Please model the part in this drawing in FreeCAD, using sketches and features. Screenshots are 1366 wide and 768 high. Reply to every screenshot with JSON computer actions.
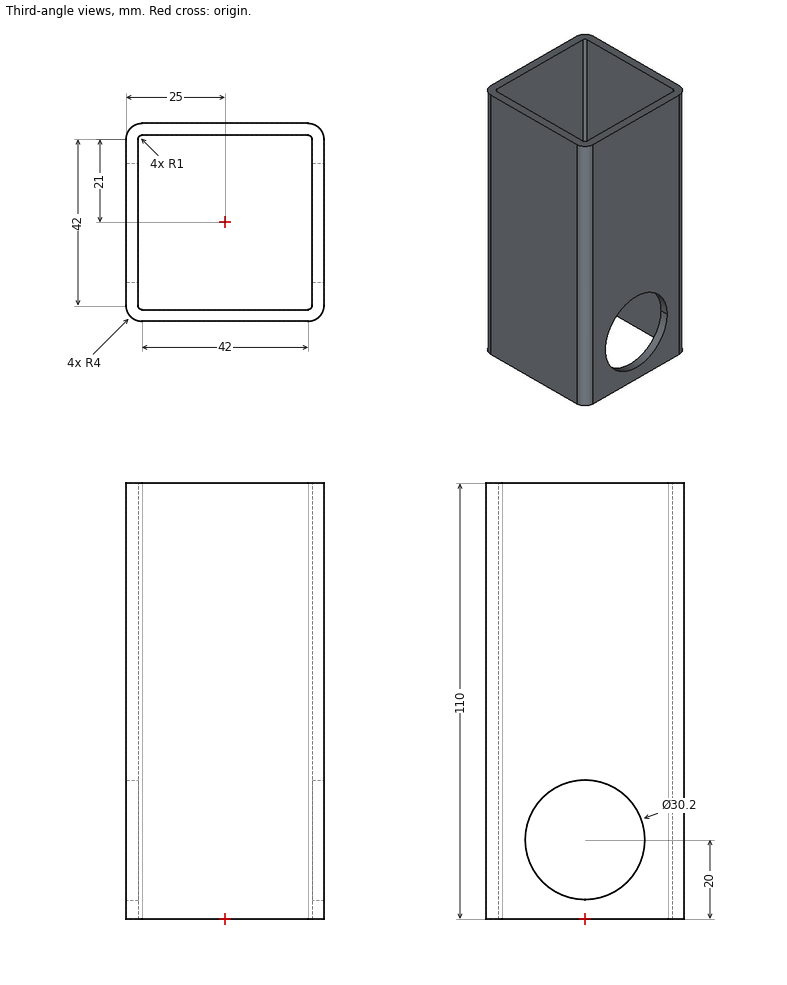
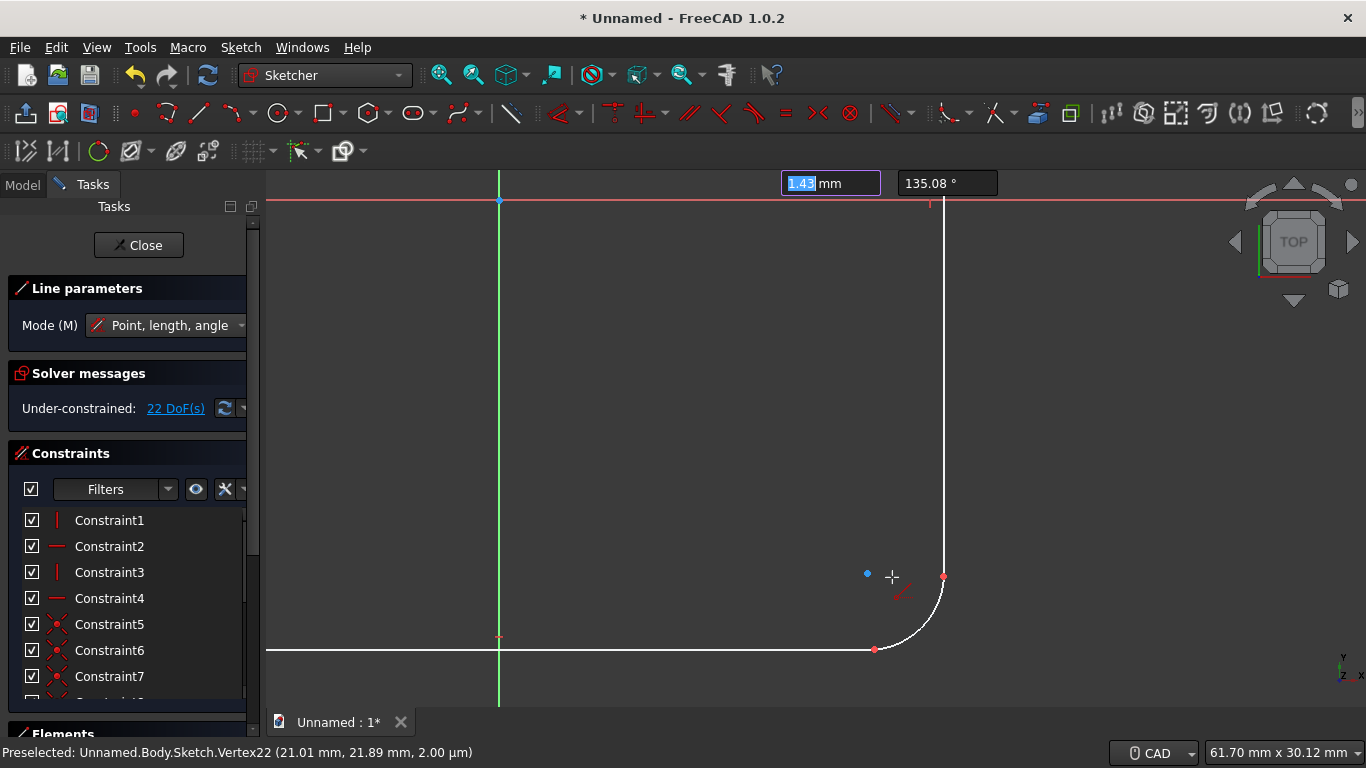
{"action": "left_click", "coordinate": [892, 574]}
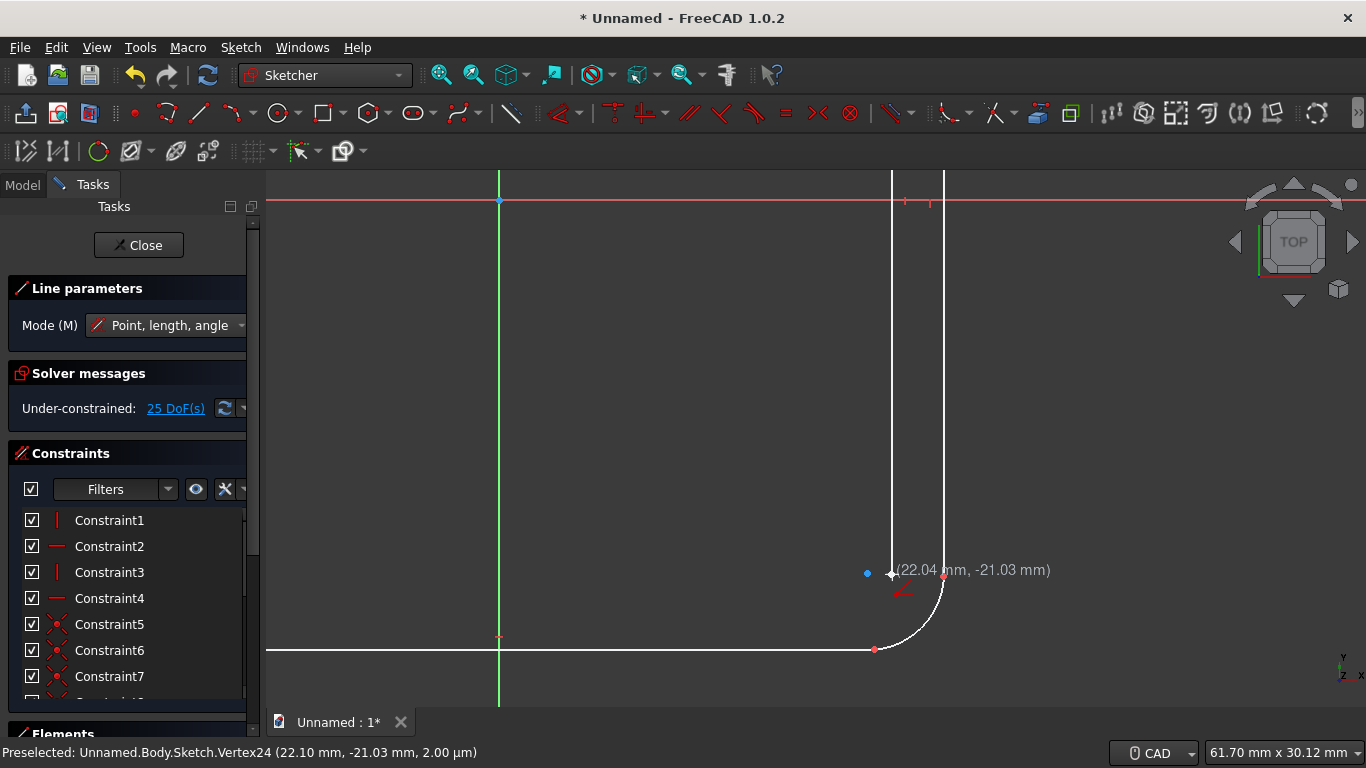
{"action": "left_click", "coordinate": [873, 592]}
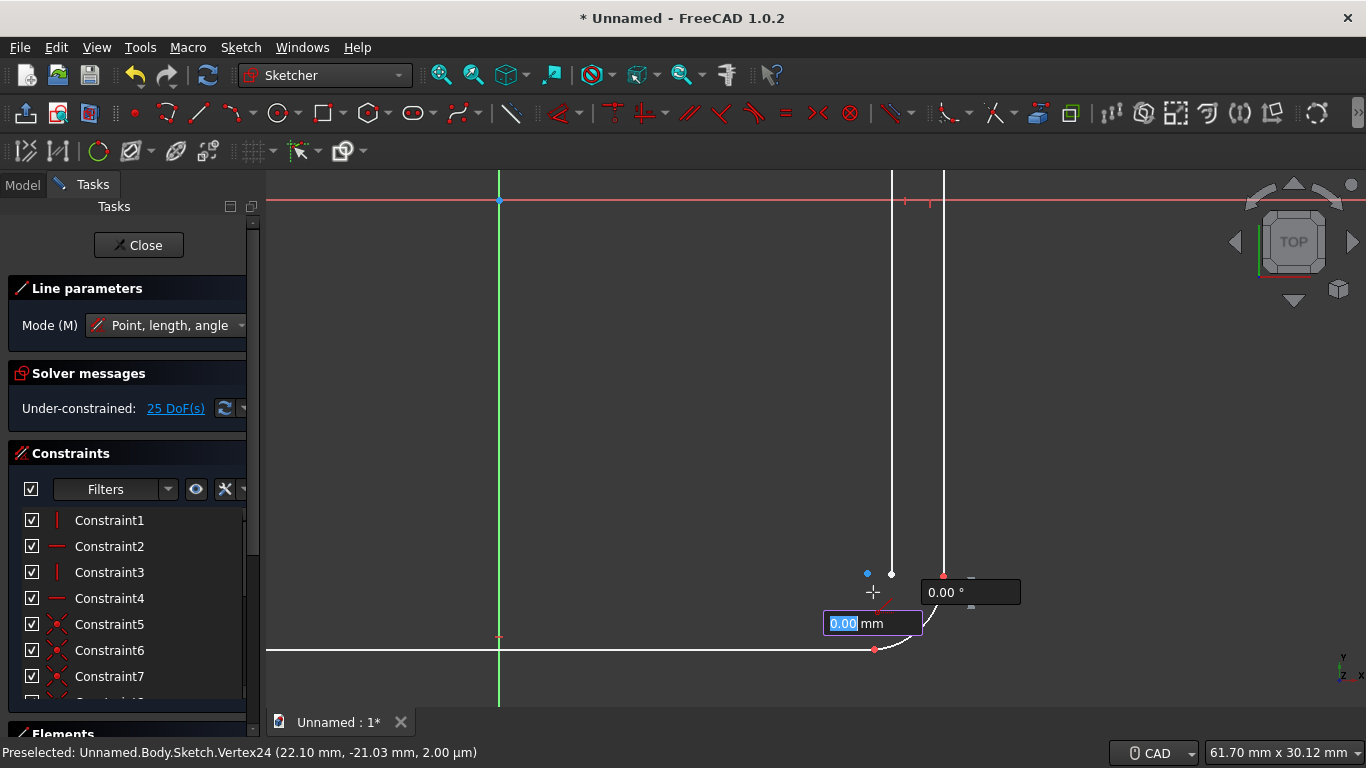
{"action": "scroll", "coordinate": [892, 577], "scroll_direction": "down", "scroll_amount": 5}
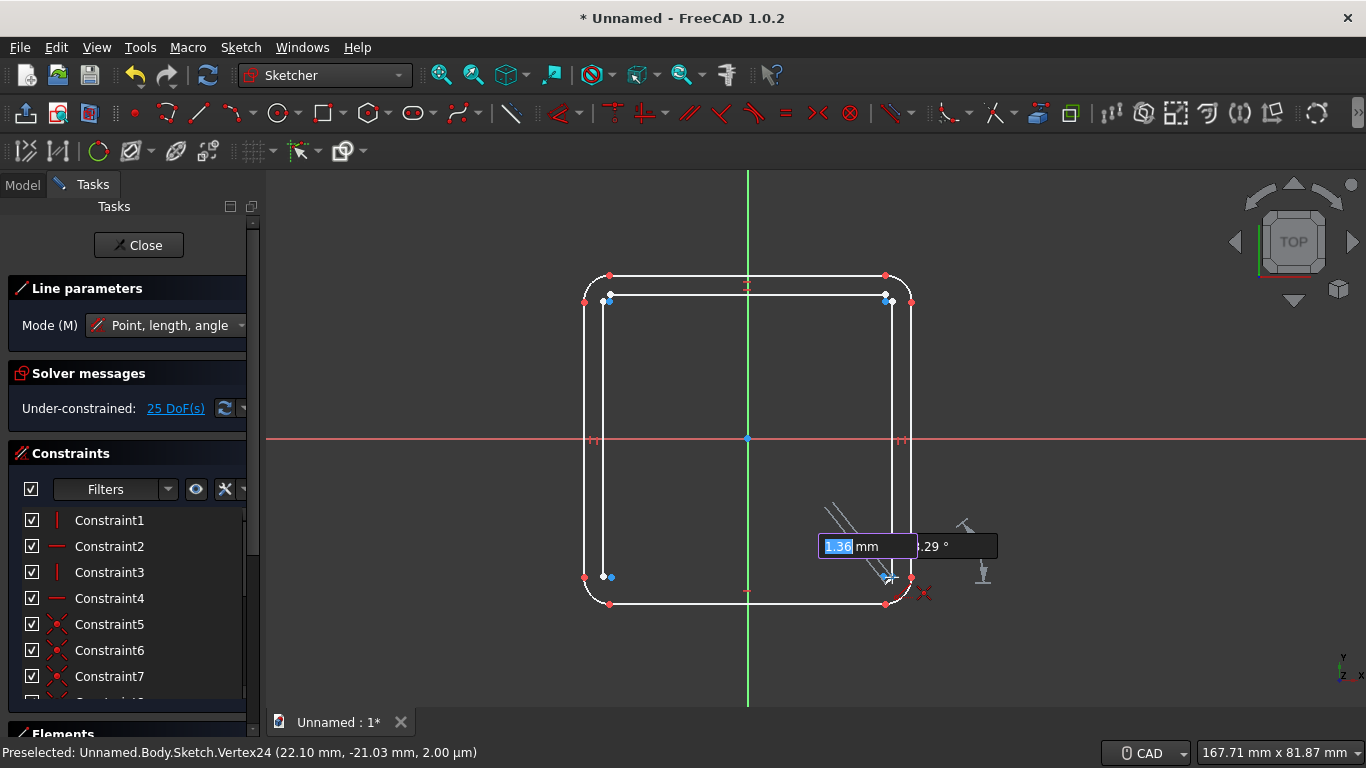
{"action": "scroll", "coordinate": [610, 583], "scroll_direction": "up", "scroll_amount": 5}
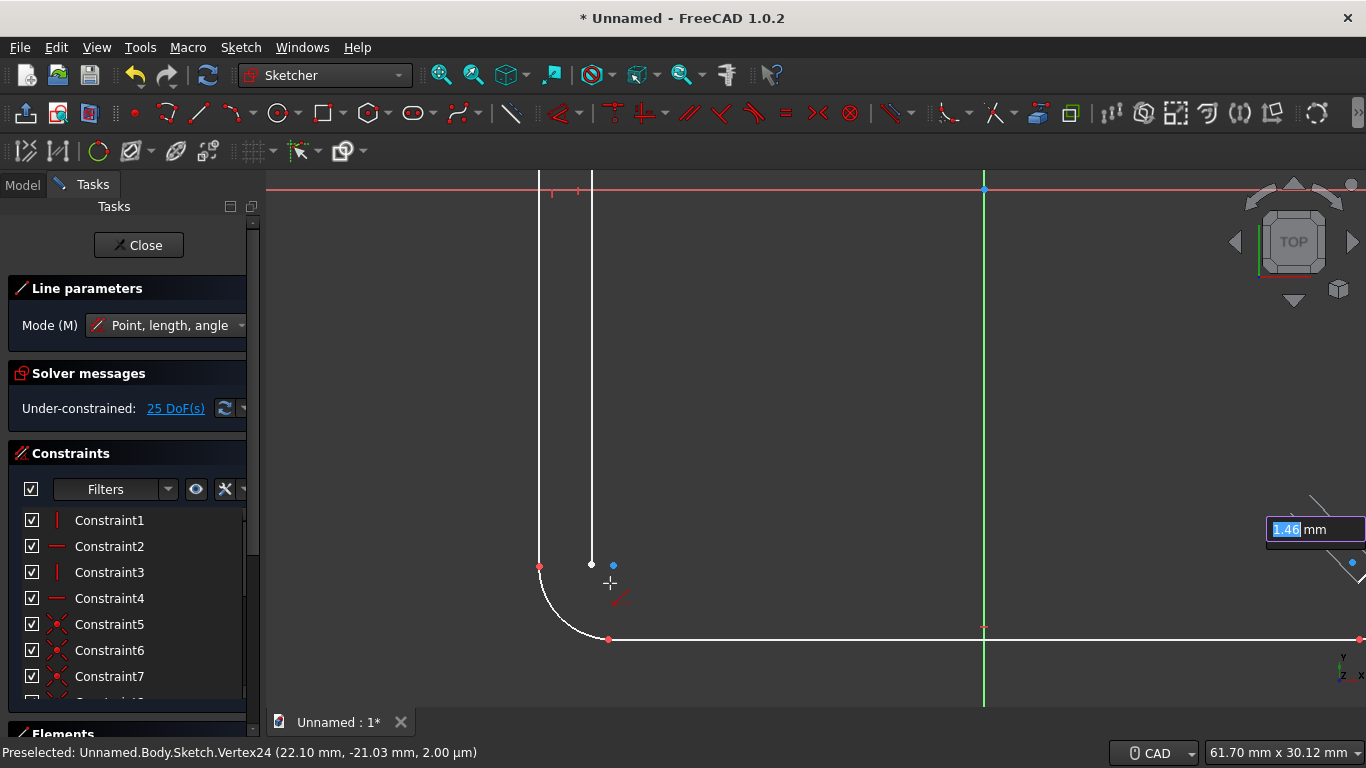
{"action": "left_click", "coordinate": [610, 582]}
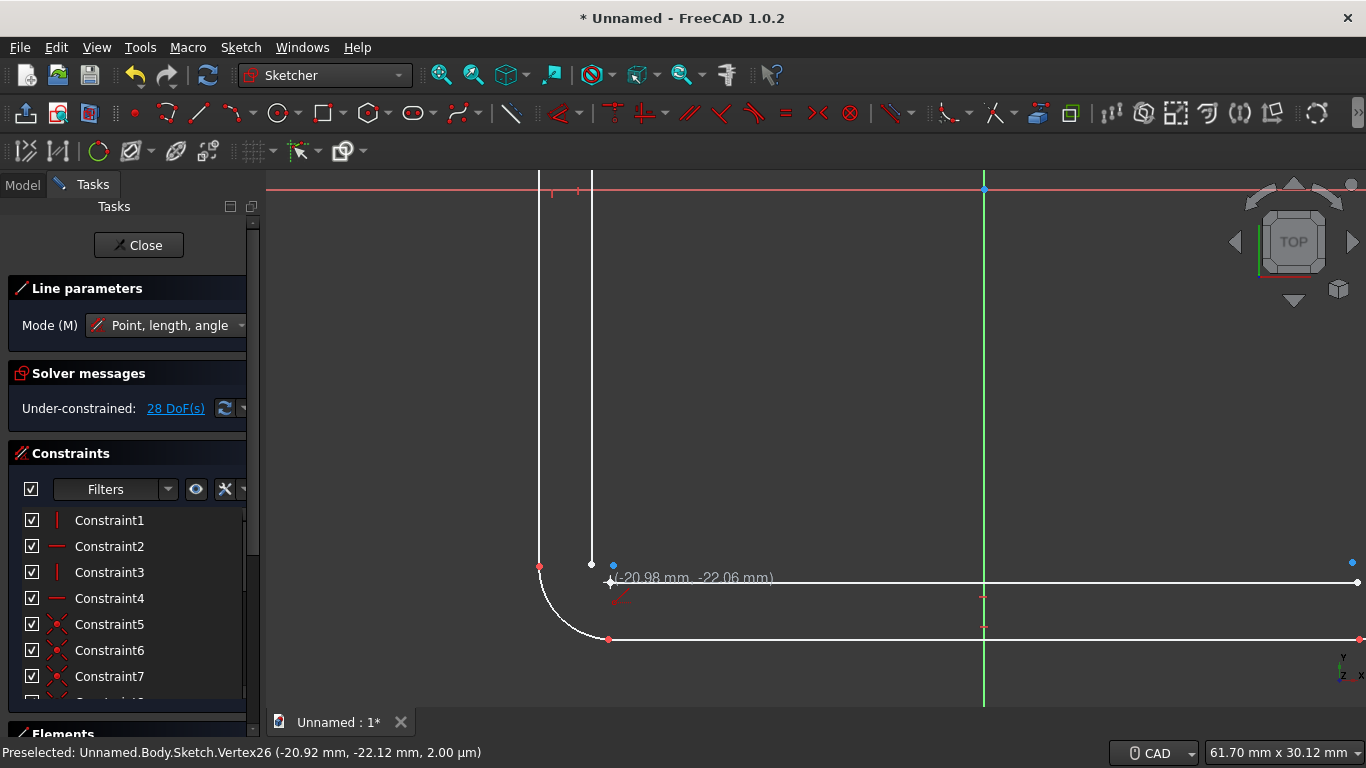
{"action": "left_click", "coordinate": [232, 114]}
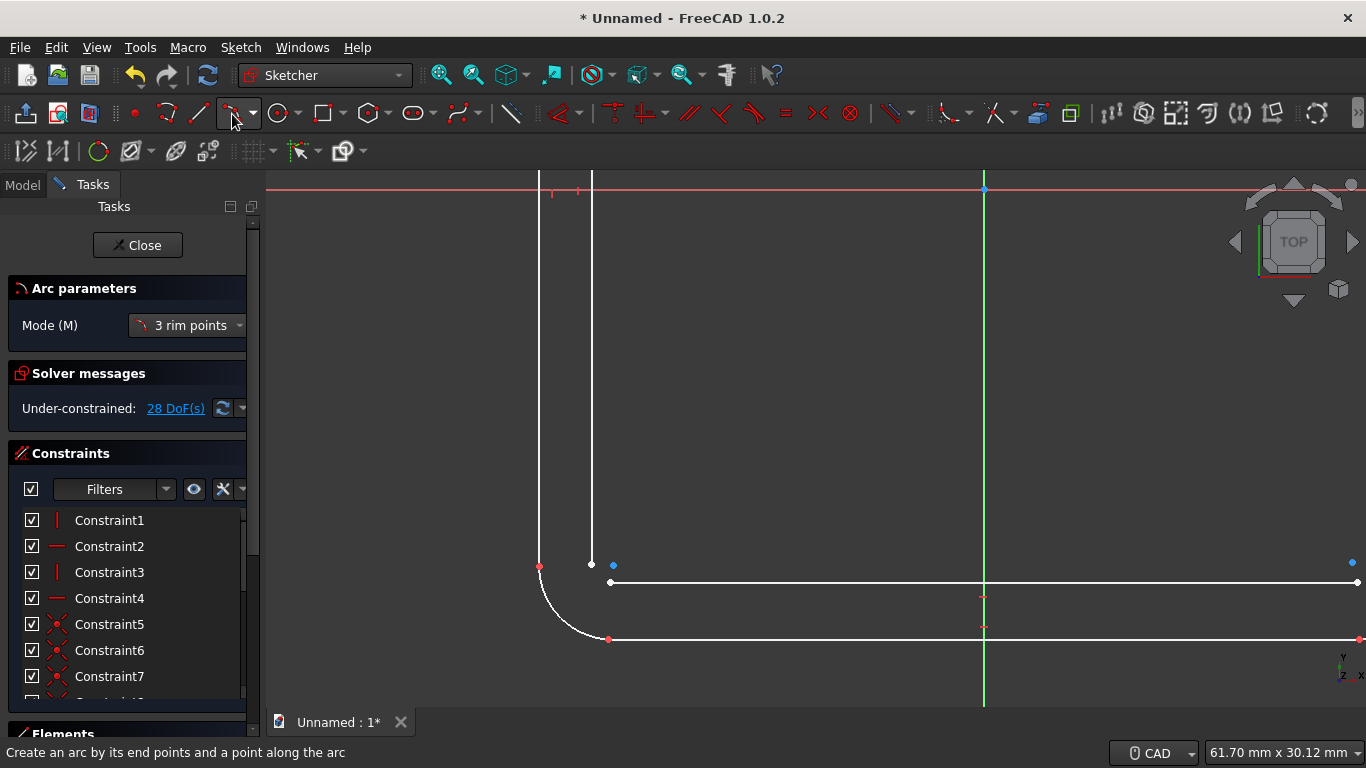
{"action": "scroll", "coordinate": [610, 583], "scroll_direction": "down", "scroll_amount": 5}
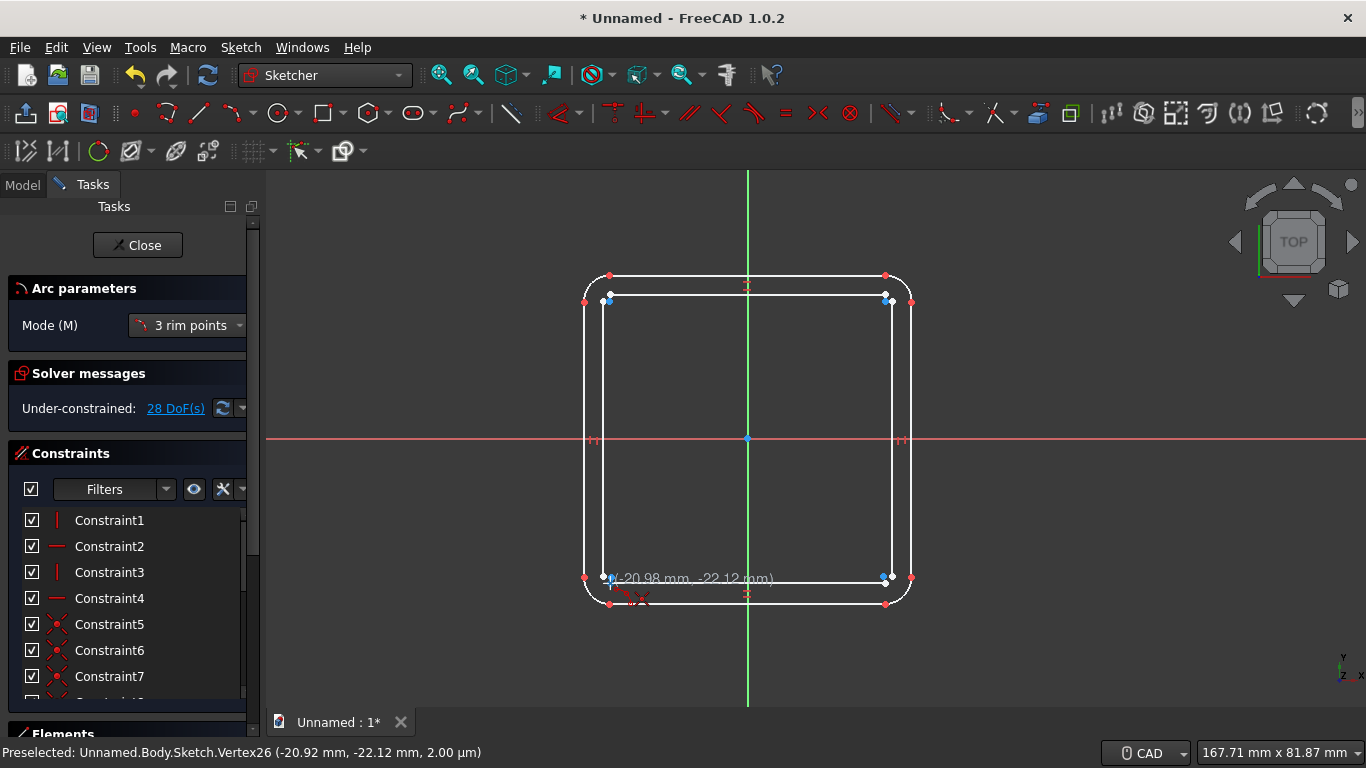
{"action": "scroll", "coordinate": [604, 301], "scroll_direction": "up", "scroll_amount": 5}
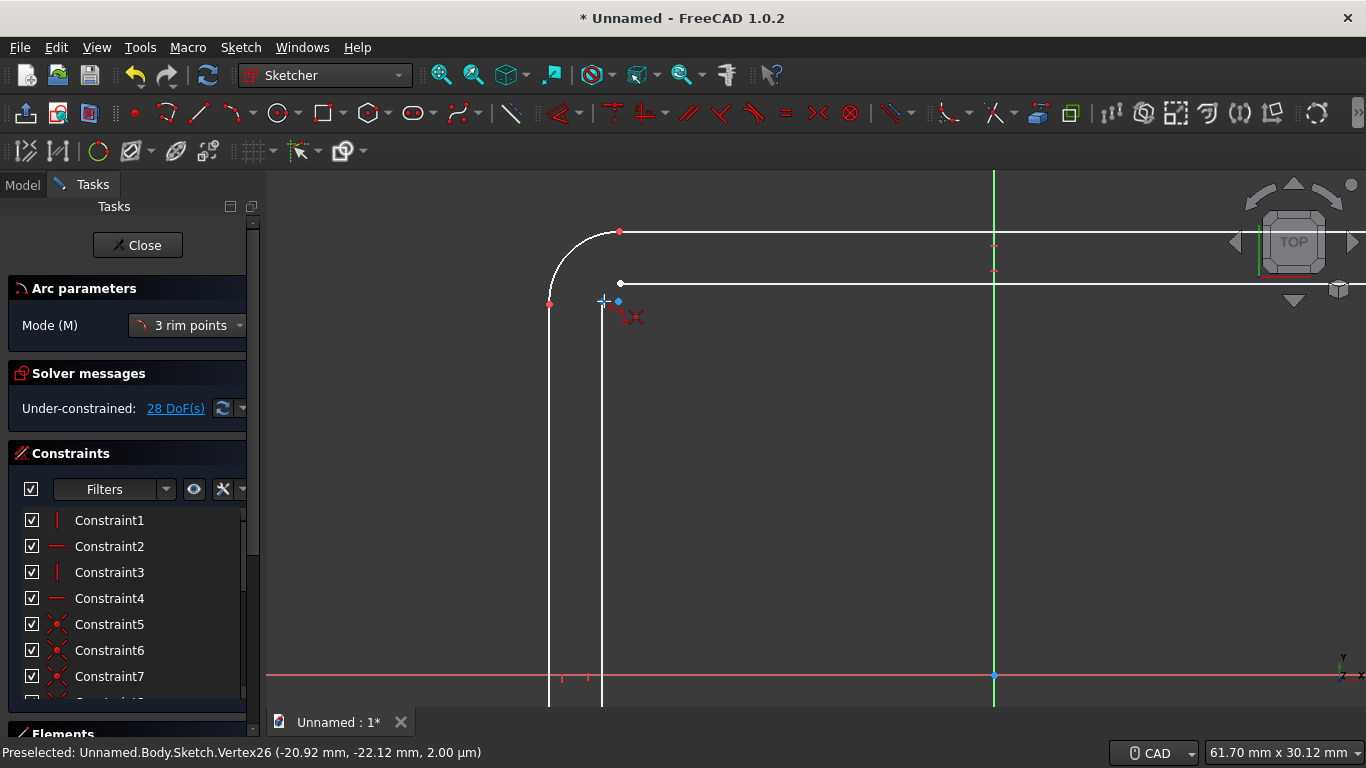
{"action": "left_click", "coordinate": [602, 302]}
{"action": "left_click", "coordinate": [620, 284]}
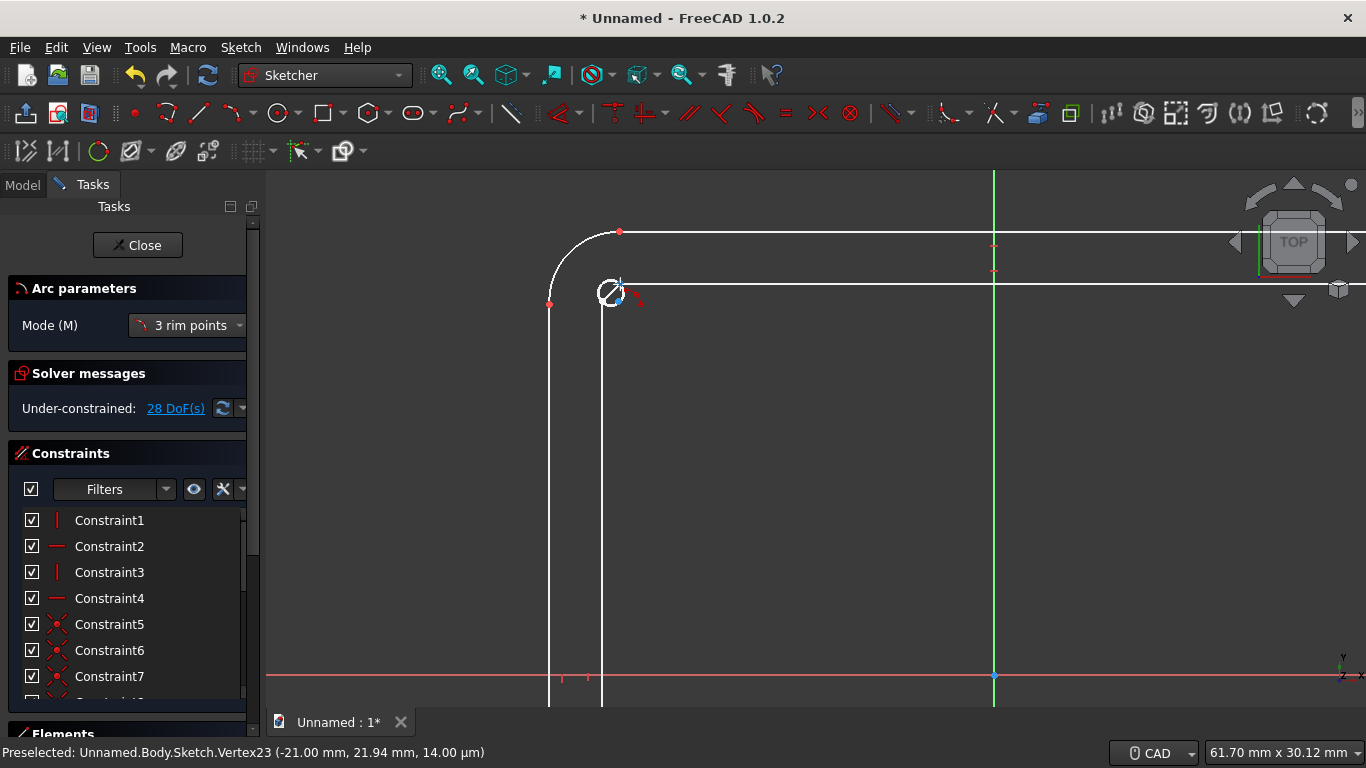
{"action": "scroll", "coordinate": [607, 288], "scroll_direction": "up", "scroll_amount": 6}